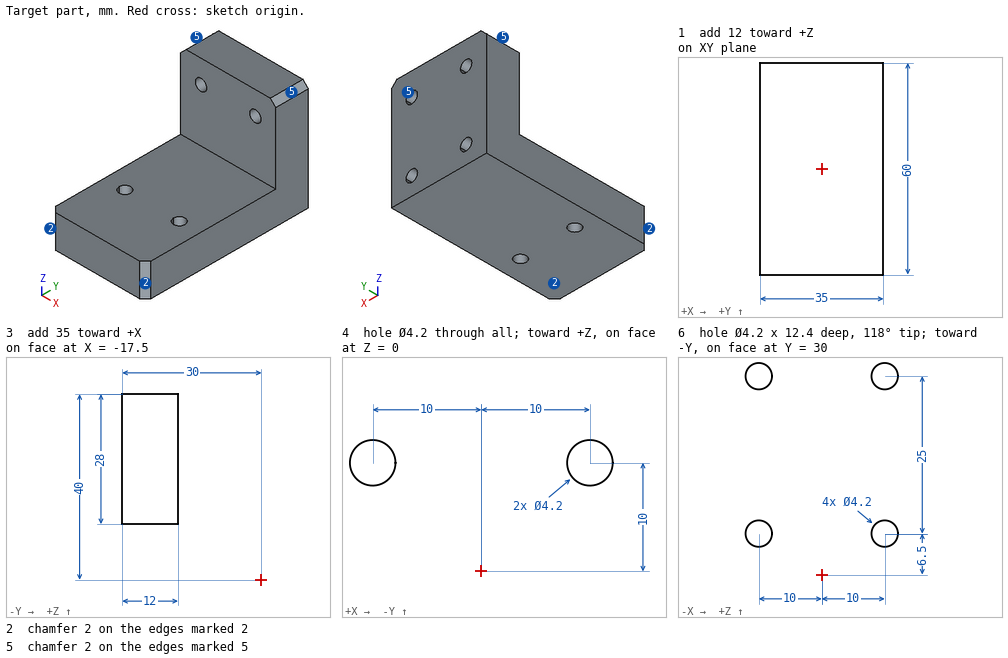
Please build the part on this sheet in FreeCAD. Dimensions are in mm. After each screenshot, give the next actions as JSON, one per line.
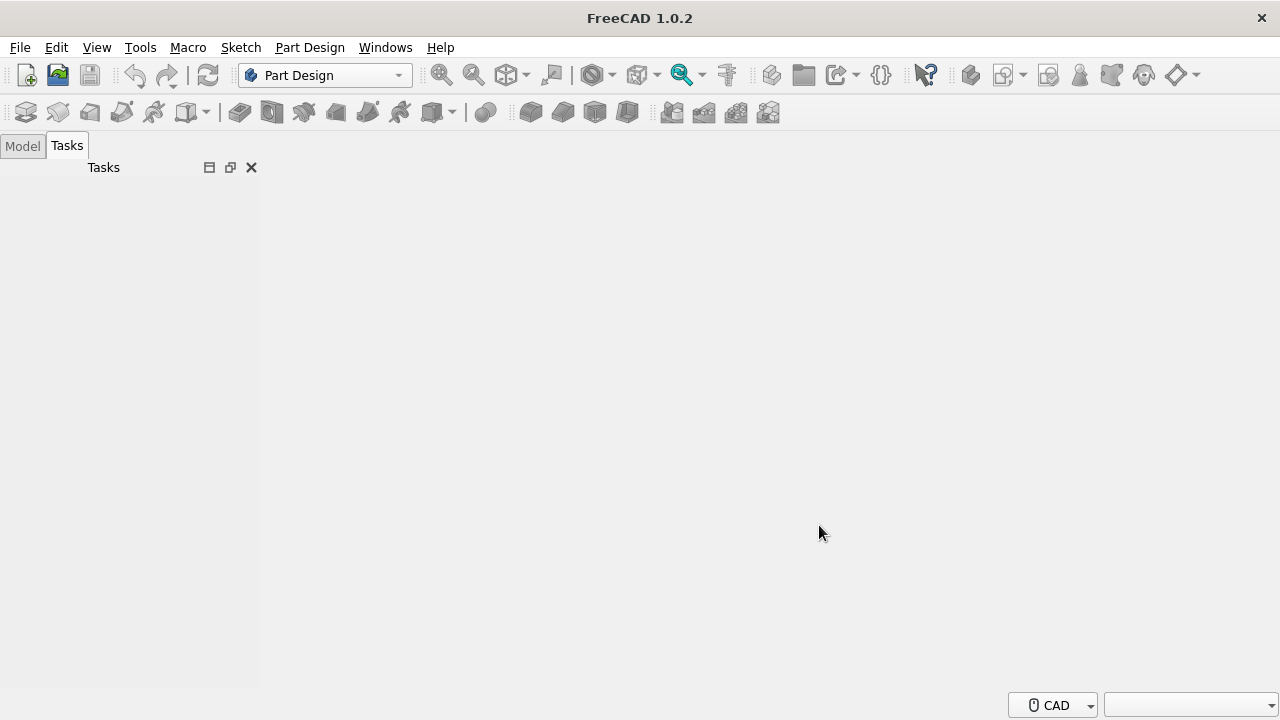
{"action": "left_click", "coordinate": [26, 76]}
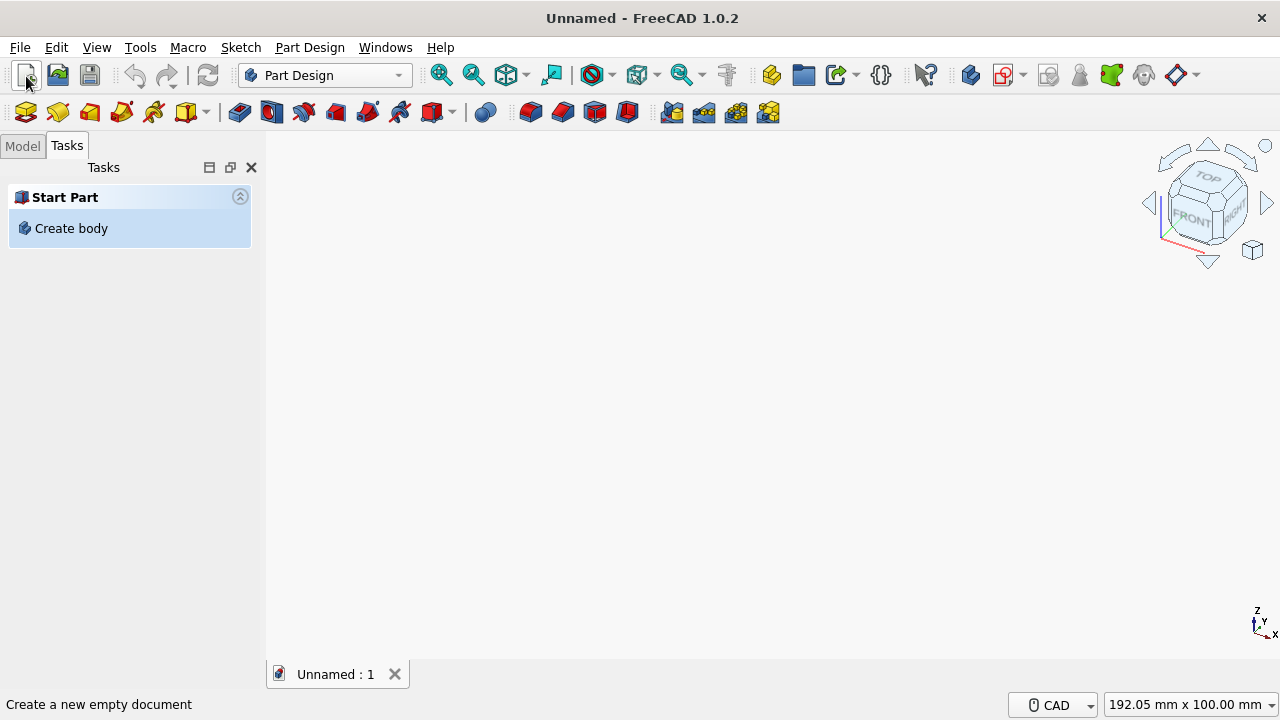
{"action": "left_click", "coordinate": [1004, 76]}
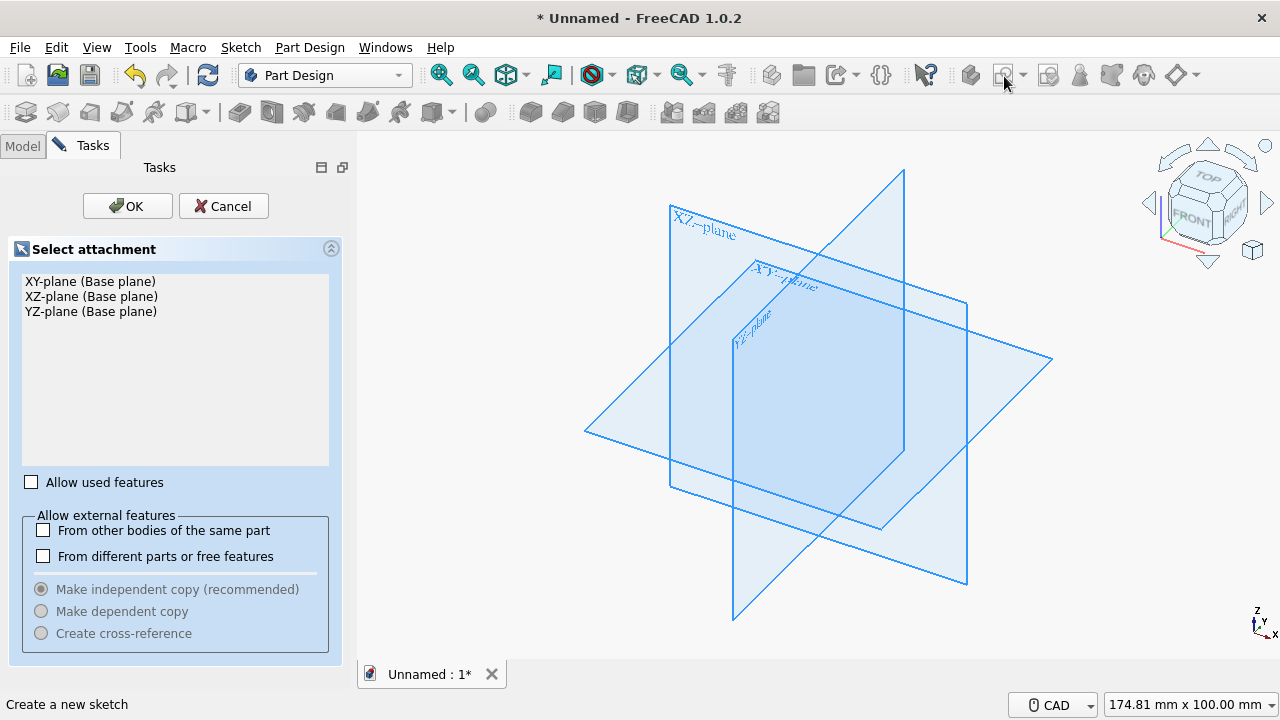
{"action": "left_click", "coordinate": [82, 282]}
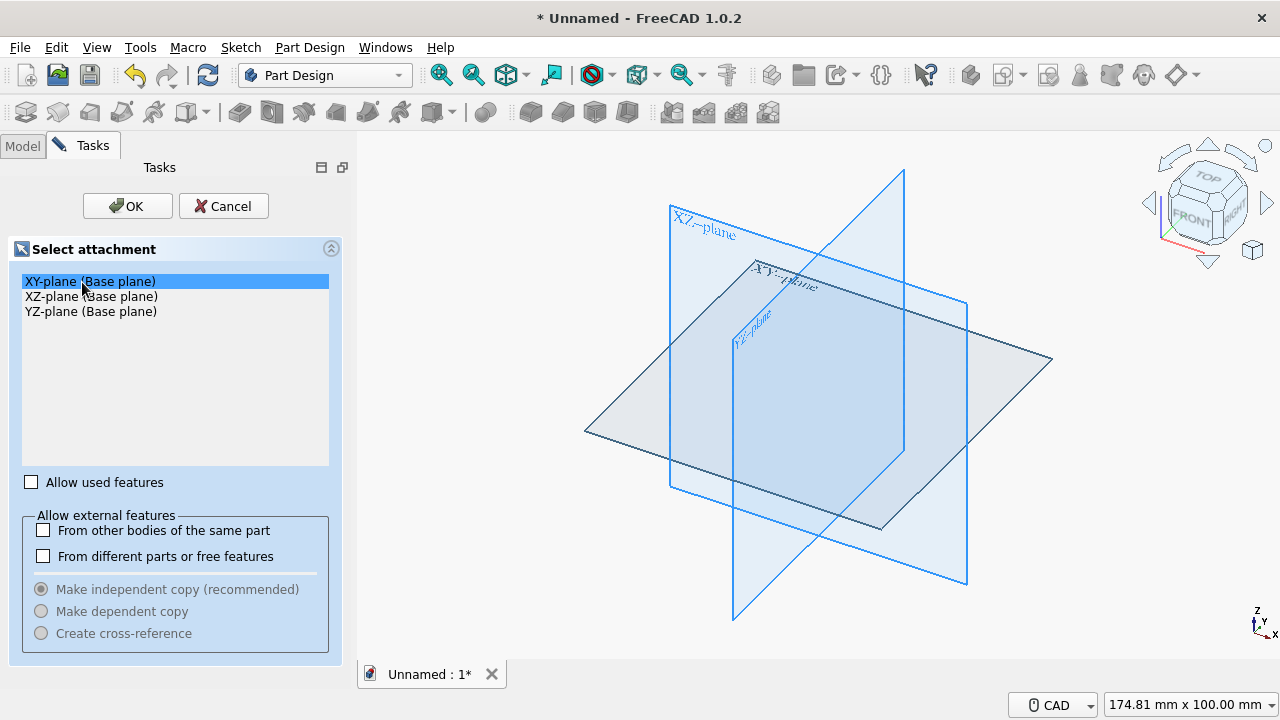
{"action": "left_click", "coordinate": [128, 206]}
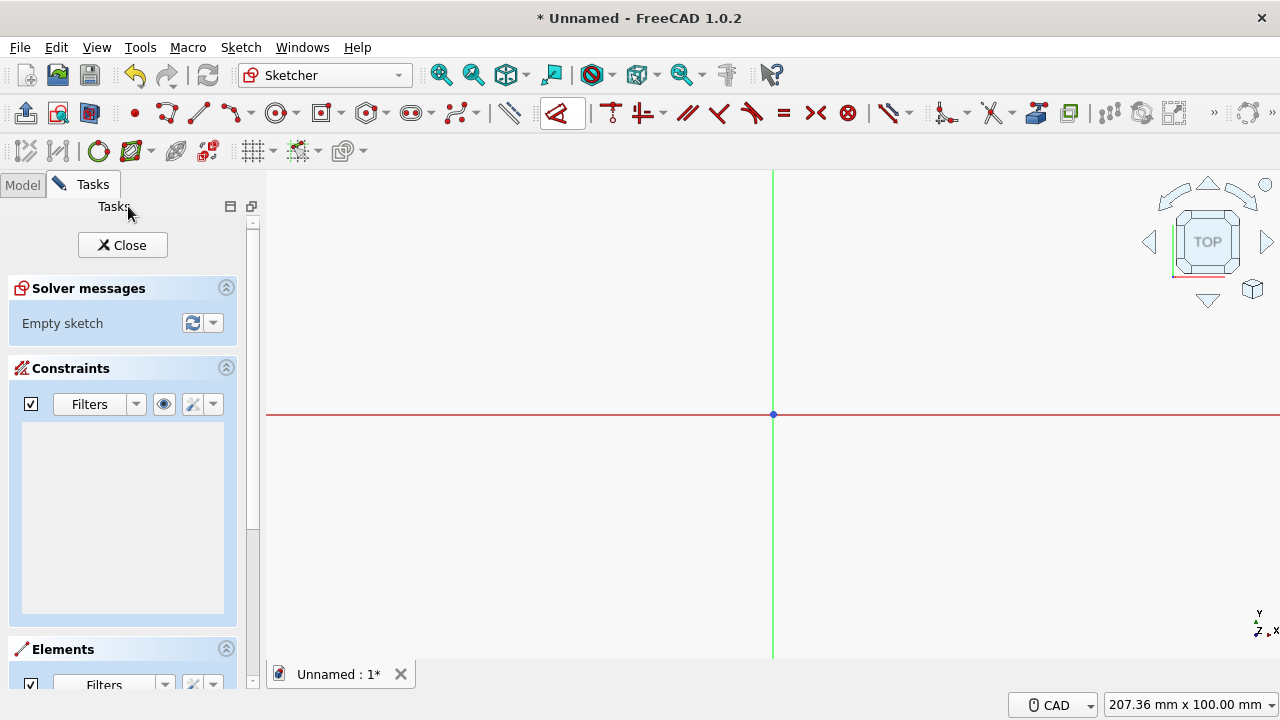
{"action": "left_click", "coordinate": [322, 114]}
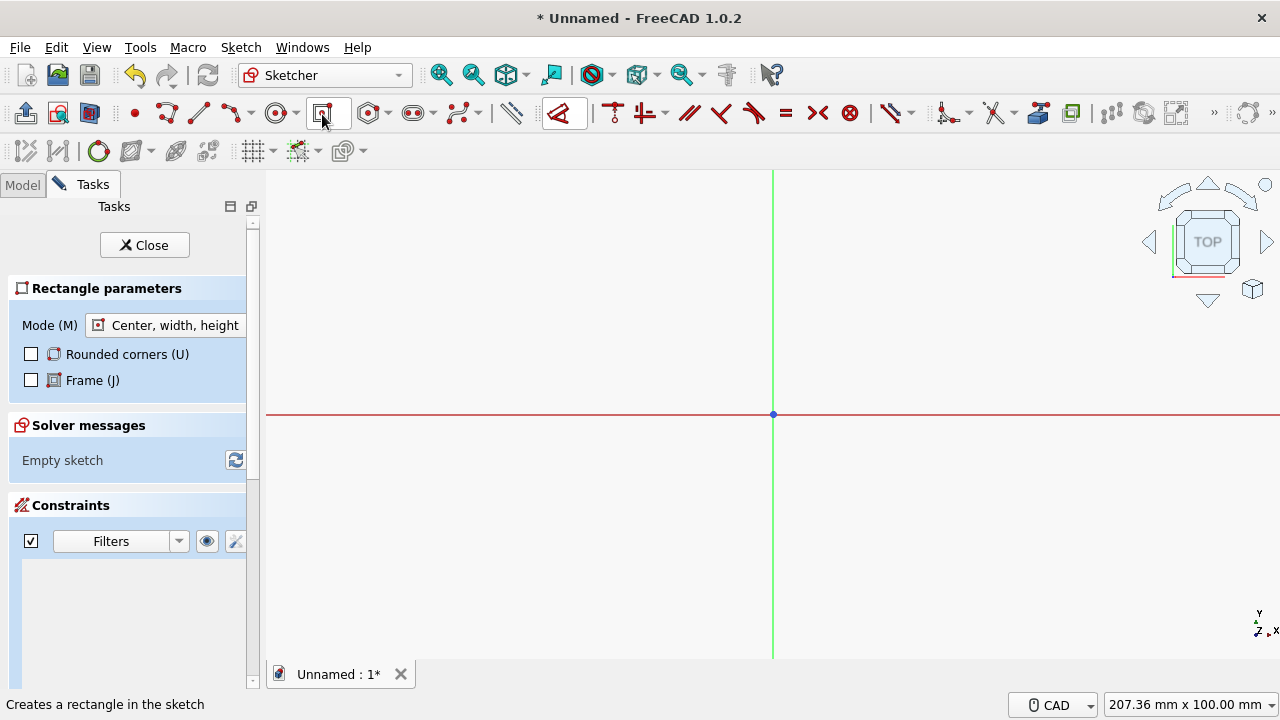
{"action": "left_click", "coordinate": [773, 414]}
{"action": "left_click", "coordinate": [859, 268]}
{"action": "key", "text": "Escape"}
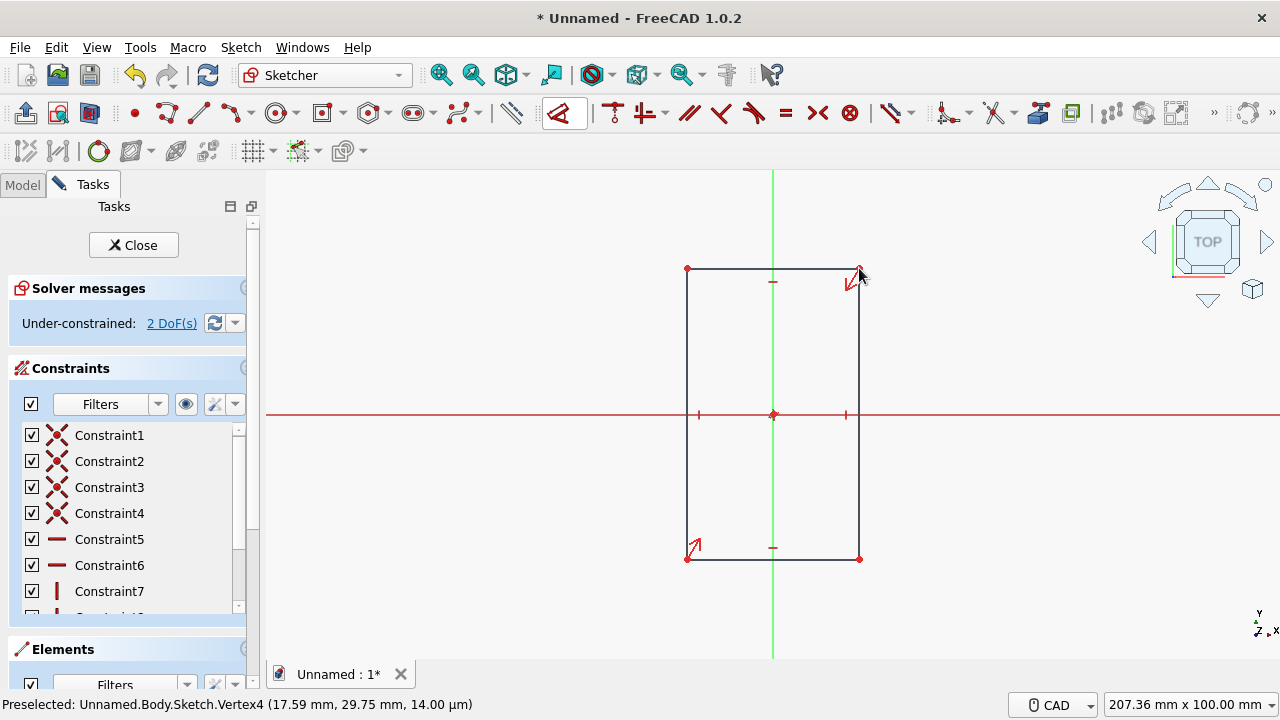
{"action": "left_click", "coordinate": [558, 114]}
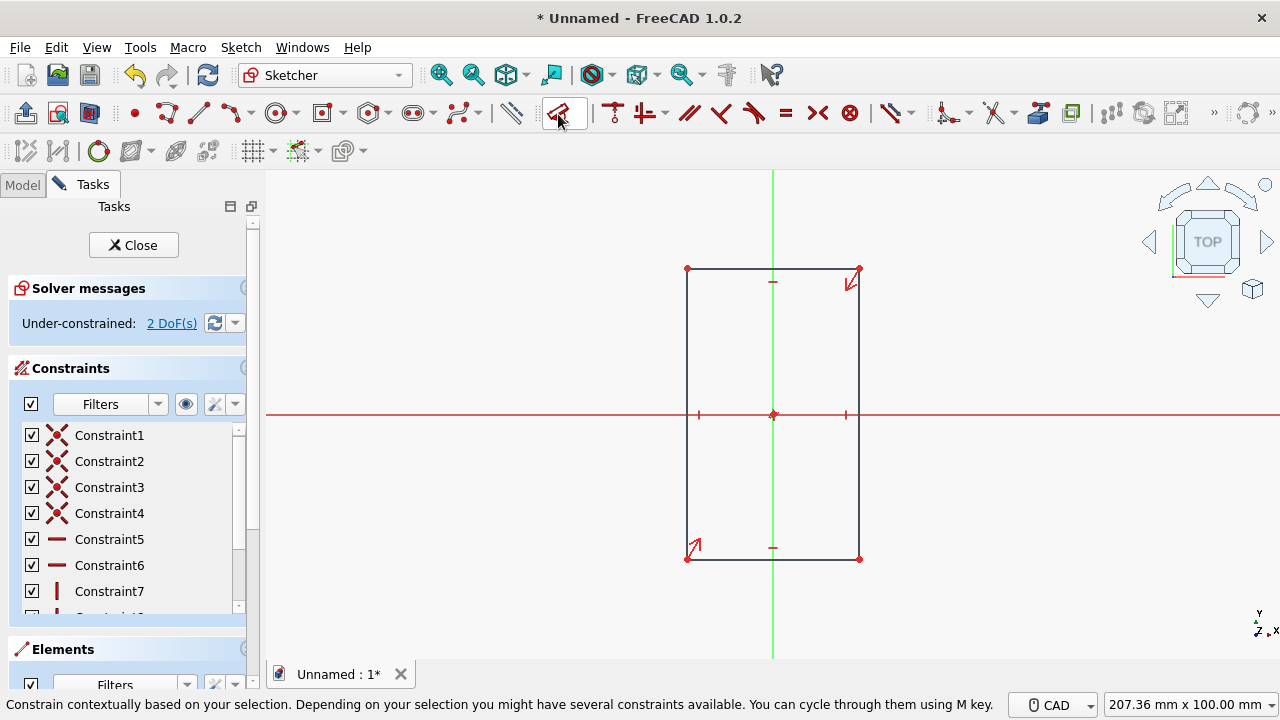
{"action": "left_click", "coordinate": [739, 560]}
{"action": "left_click", "coordinate": [733, 594]}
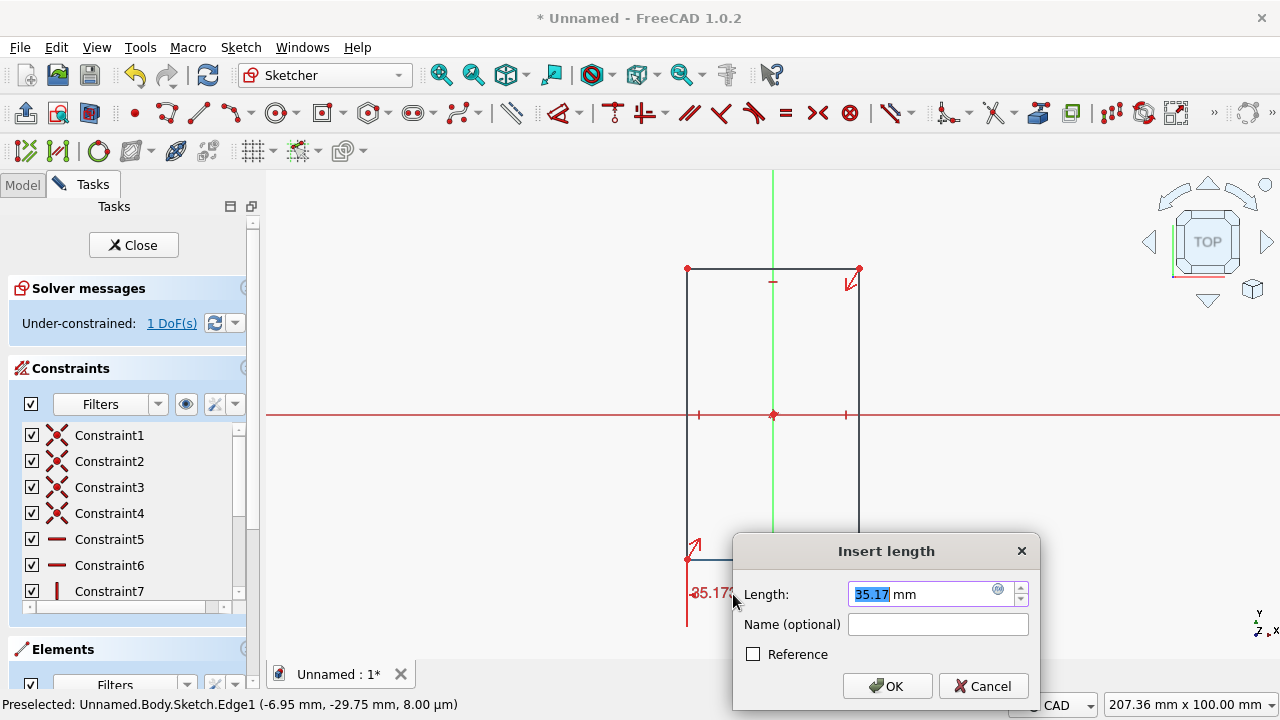
{"action": "type", "text": "35"}
{"action": "key", "text": "Return"}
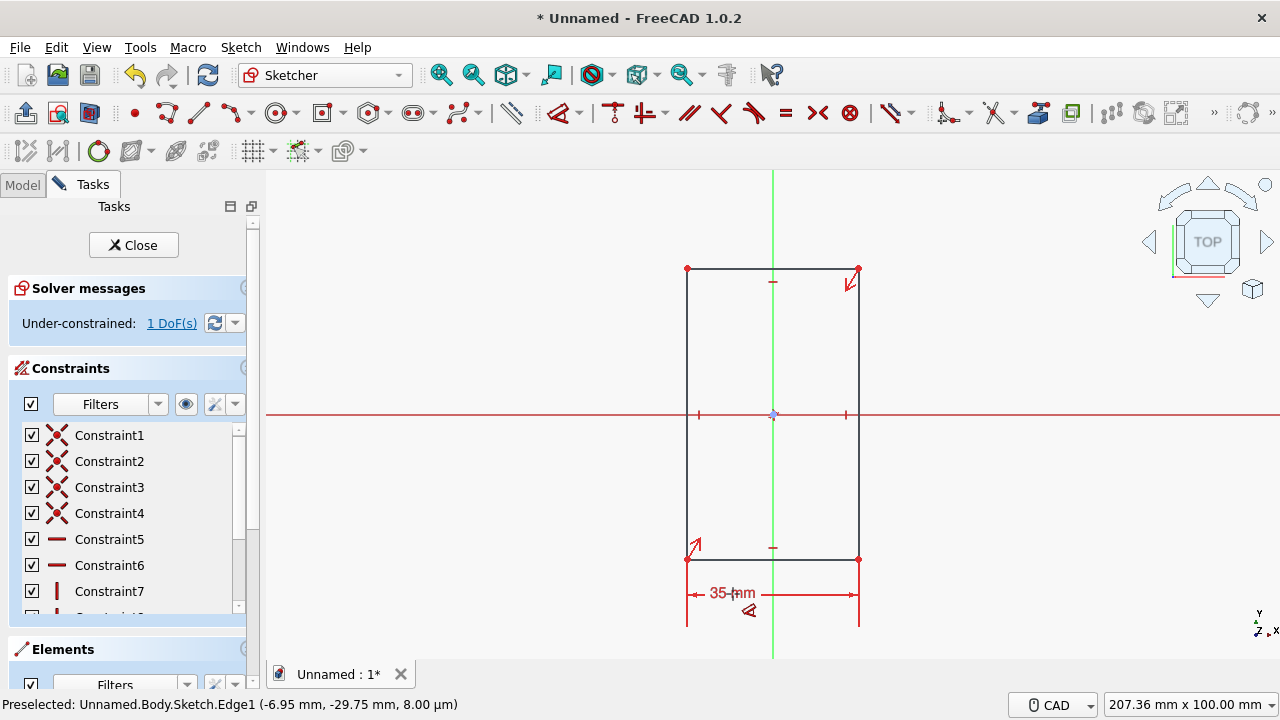
{"action": "left_click", "coordinate": [859, 473]}
{"action": "left_click", "coordinate": [893, 348]}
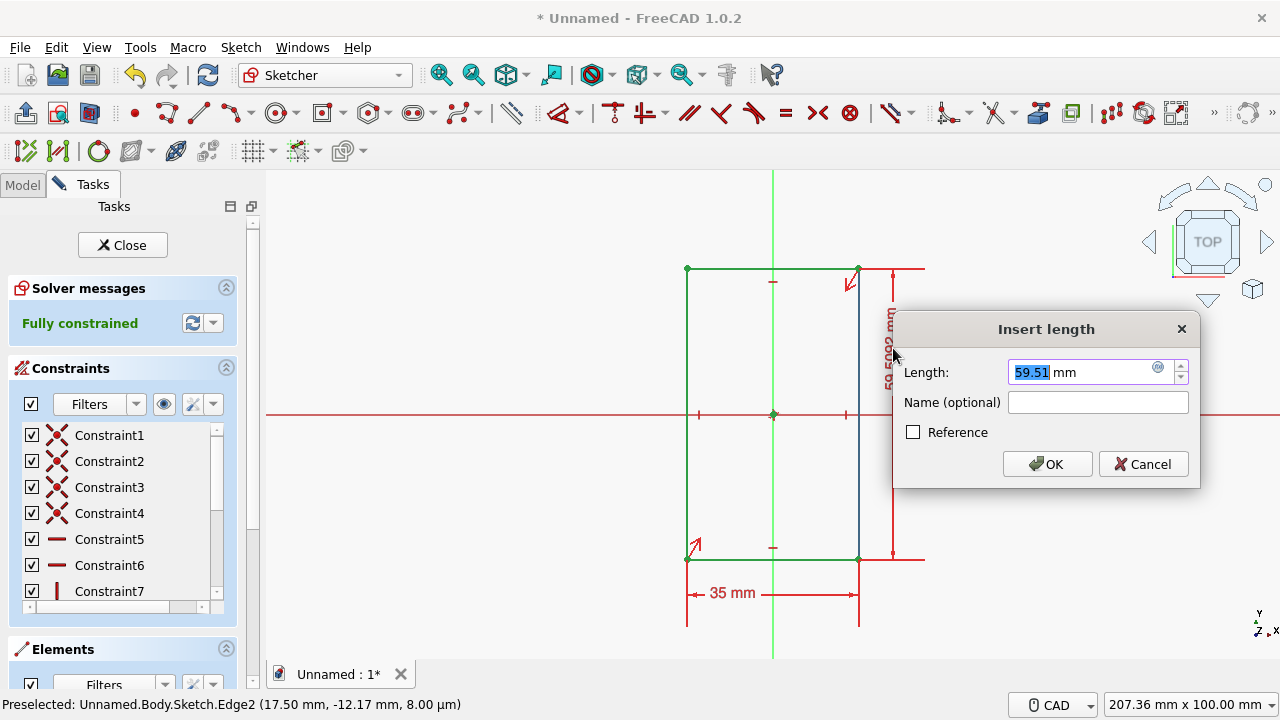
{"action": "type", "text": "60"}
{"action": "key", "text": "Return"}
{"action": "key", "text": "Escape"}